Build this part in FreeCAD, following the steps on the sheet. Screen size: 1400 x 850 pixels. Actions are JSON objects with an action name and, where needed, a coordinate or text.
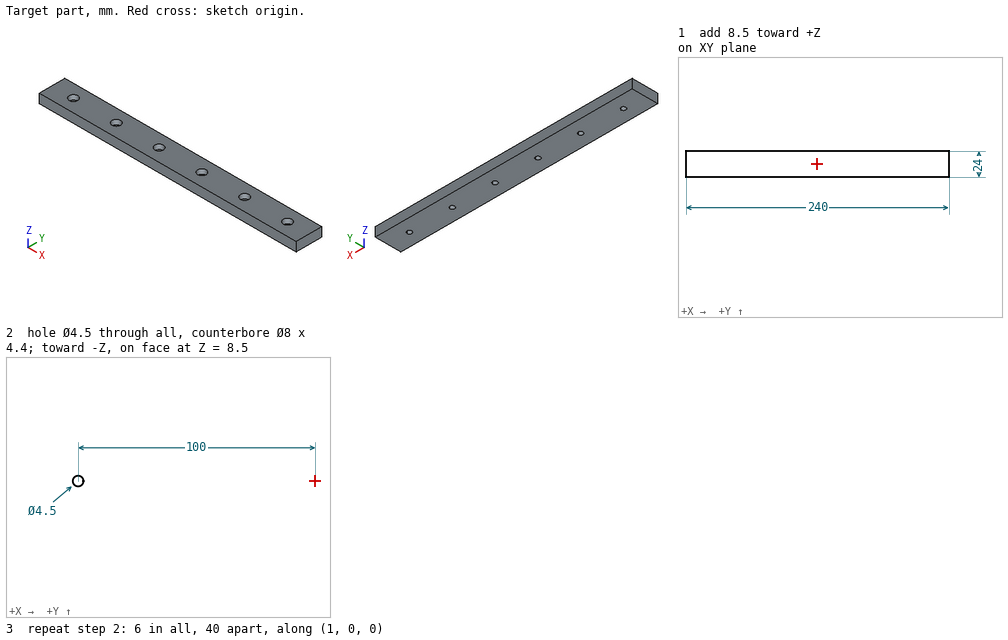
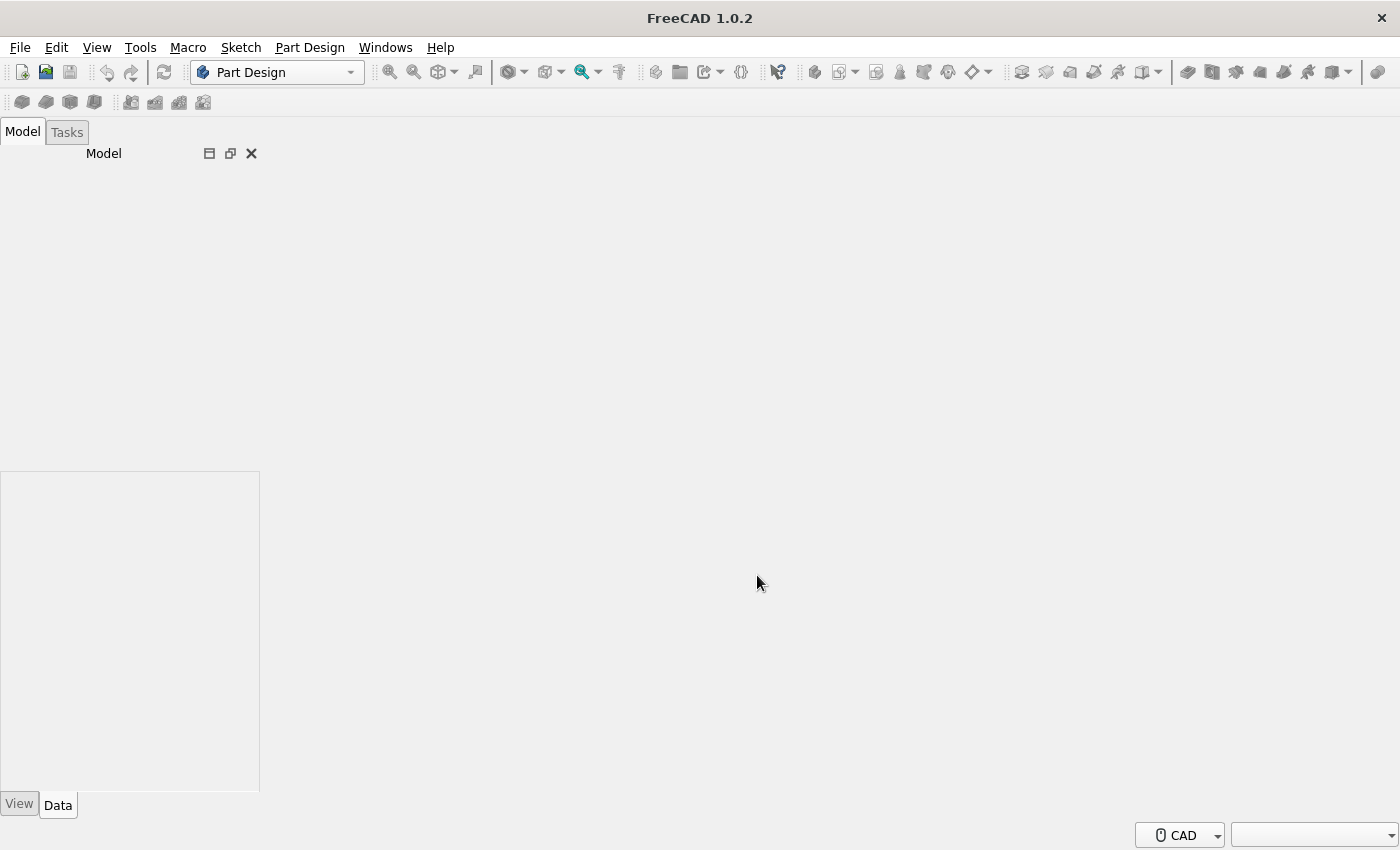
{"action": "key", "text": "ctrl+n"}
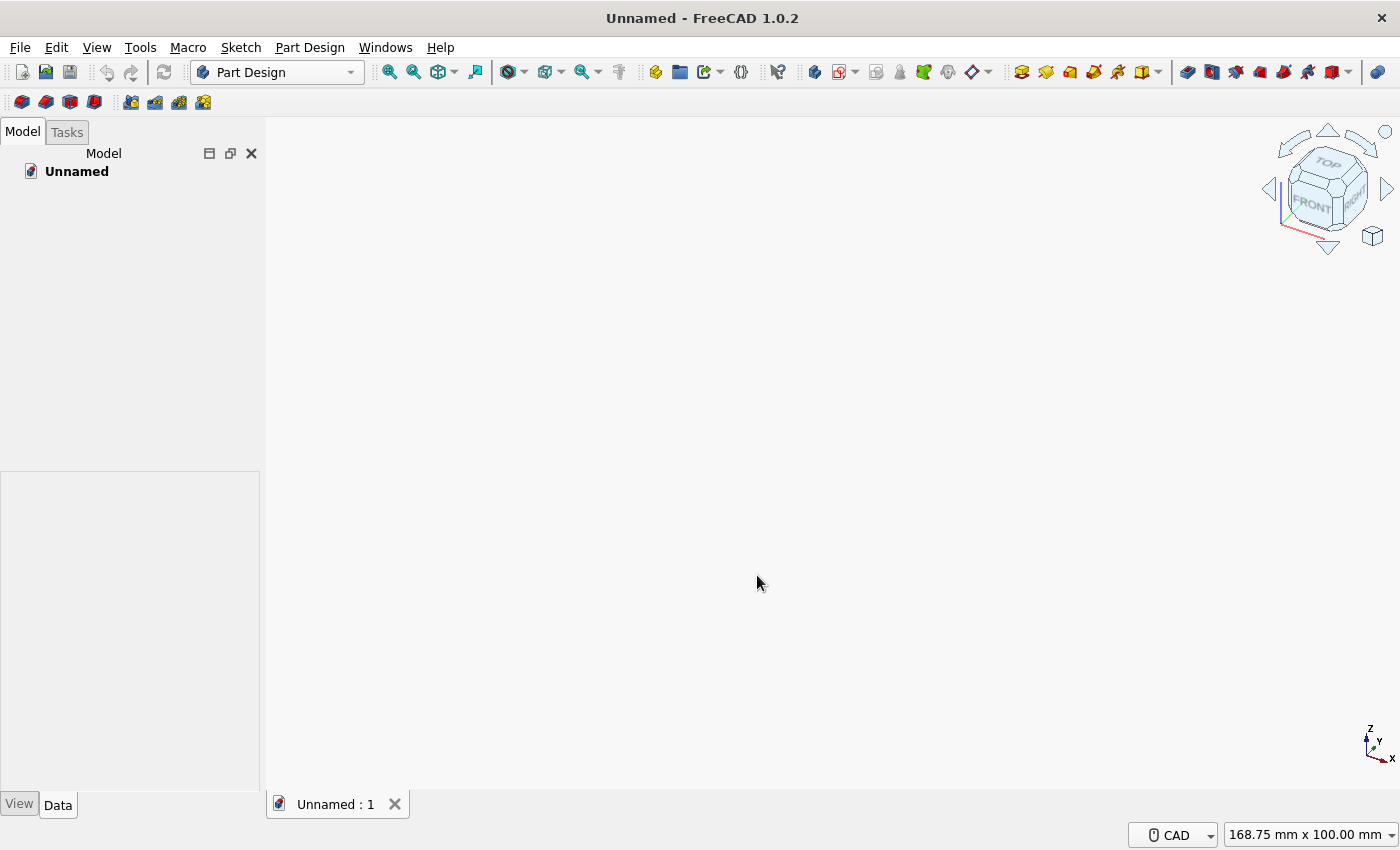
{"action": "left_click", "coordinate": [840, 72]}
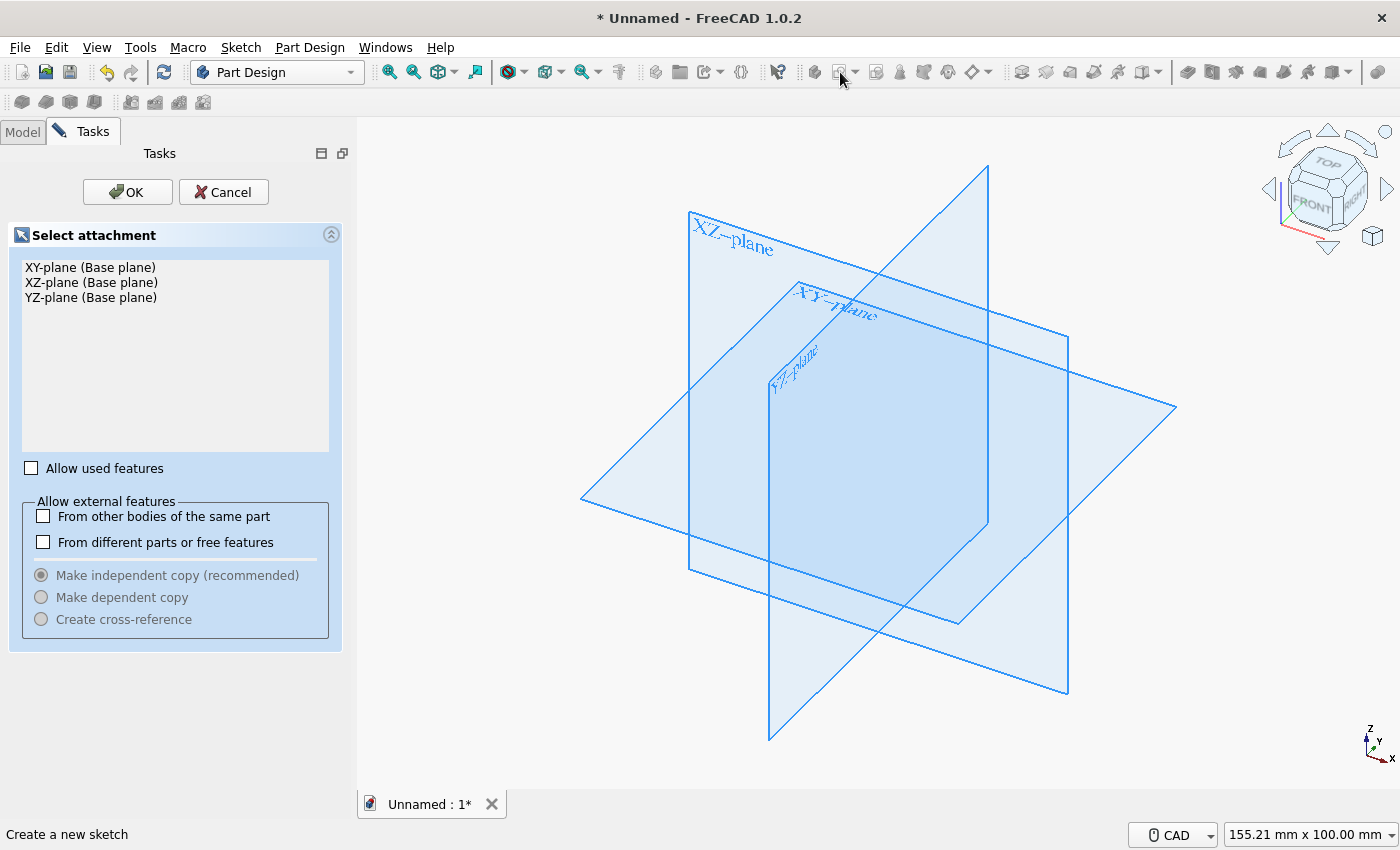
{"action": "left_click", "coordinate": [82, 268]}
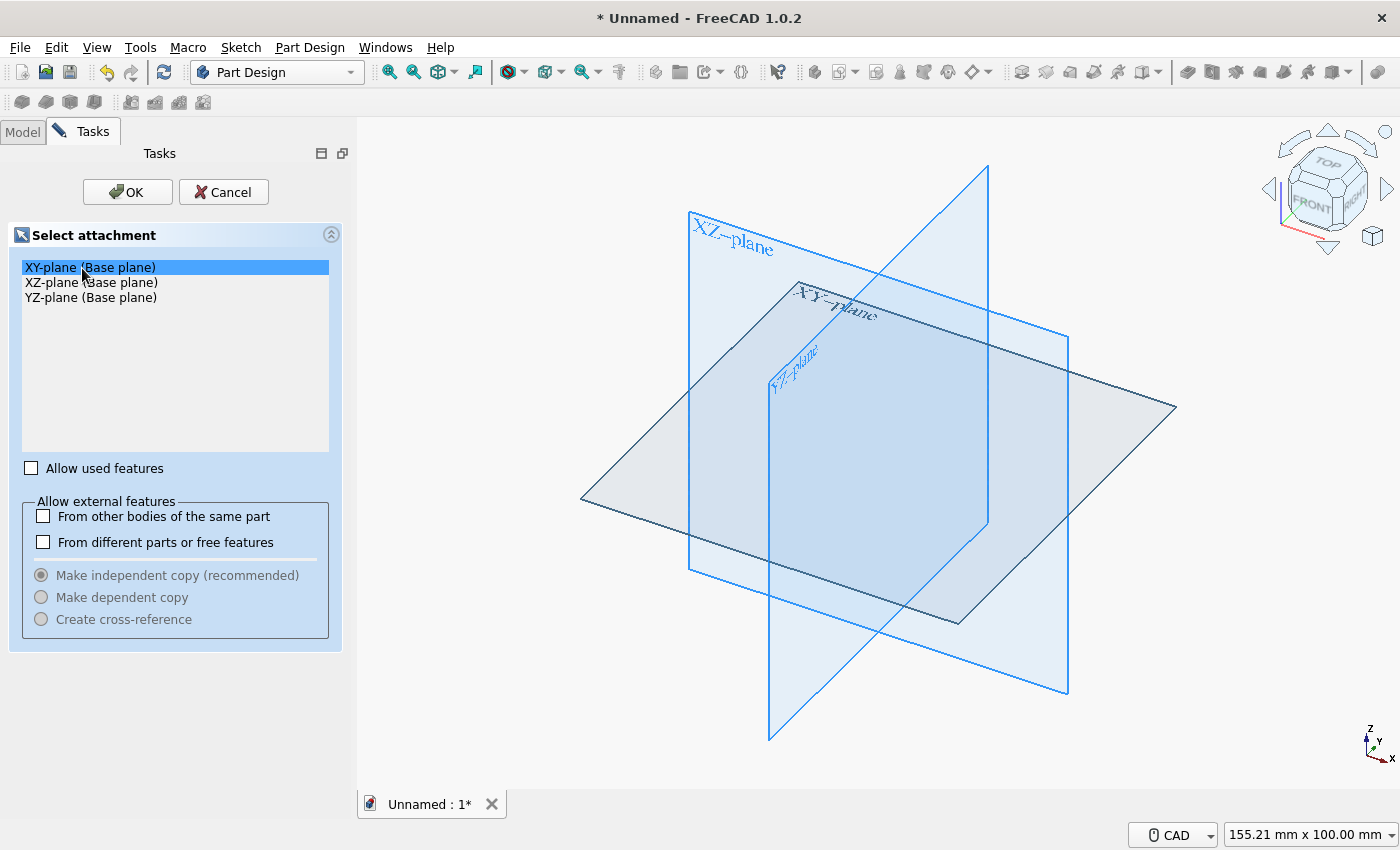
{"action": "left_click", "coordinate": [128, 192]}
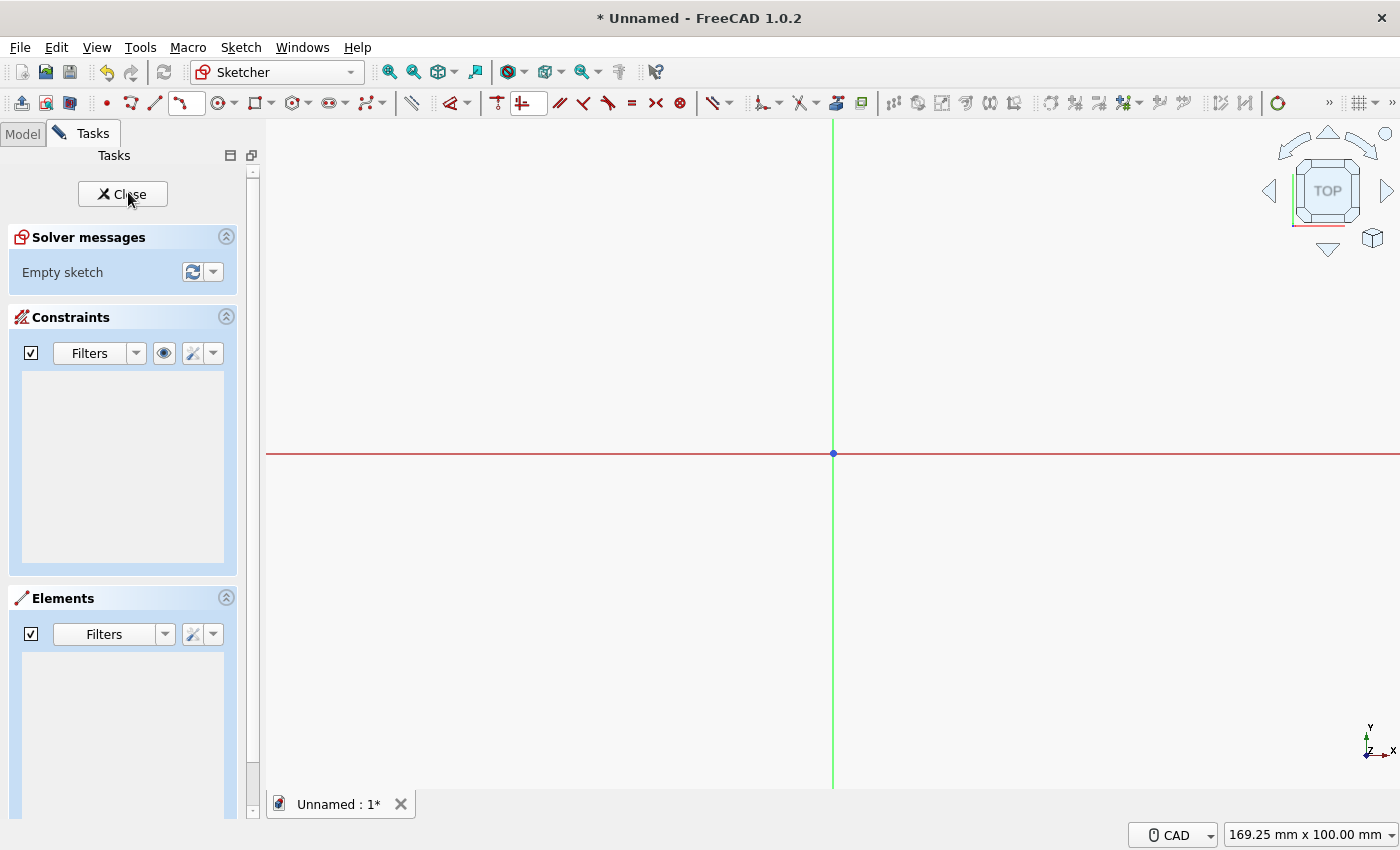
{"action": "scroll", "coordinate": [709, 454], "scroll_direction": "down", "scroll_amount": 4}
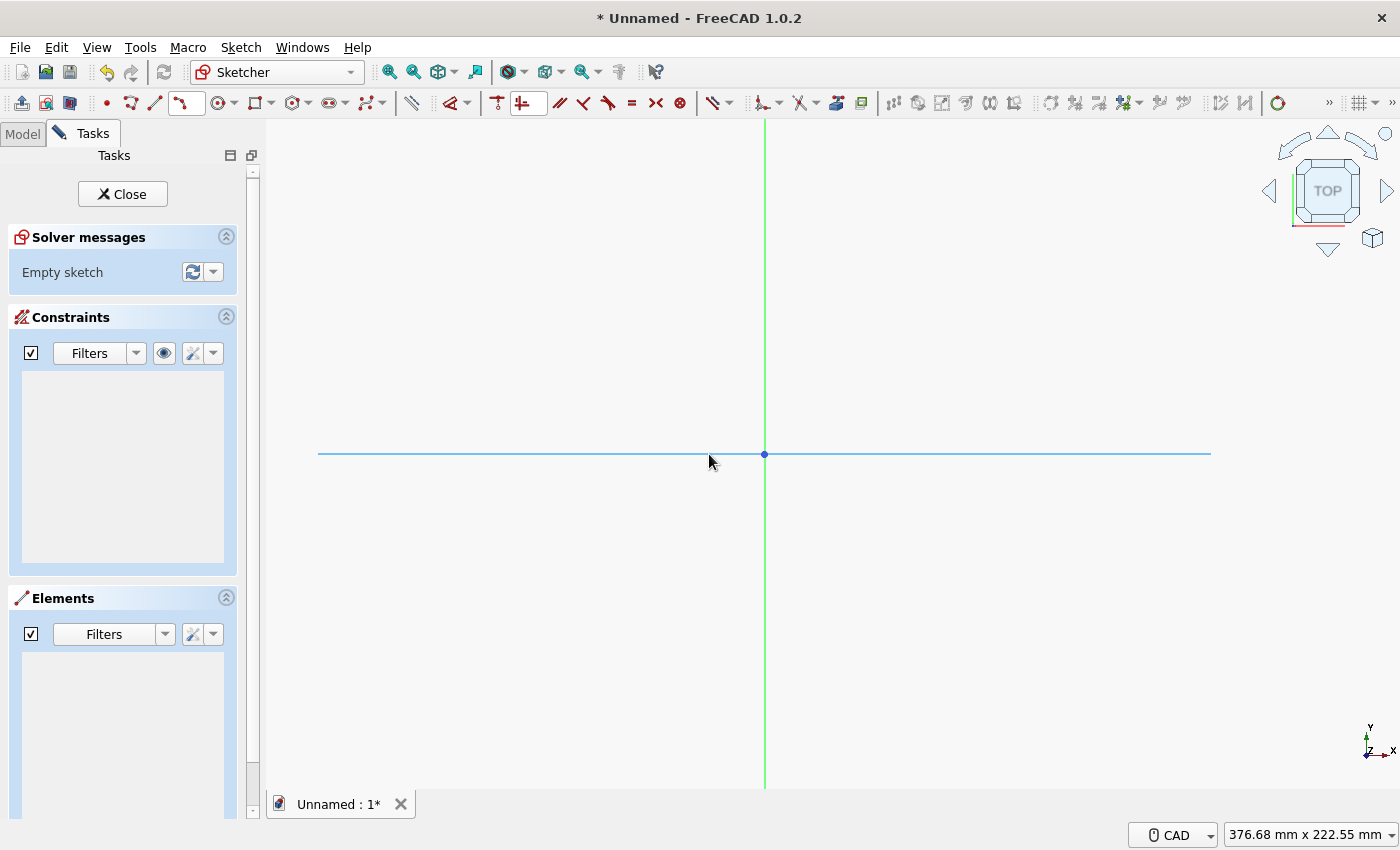
{"action": "left_click", "coordinate": [274, 104]}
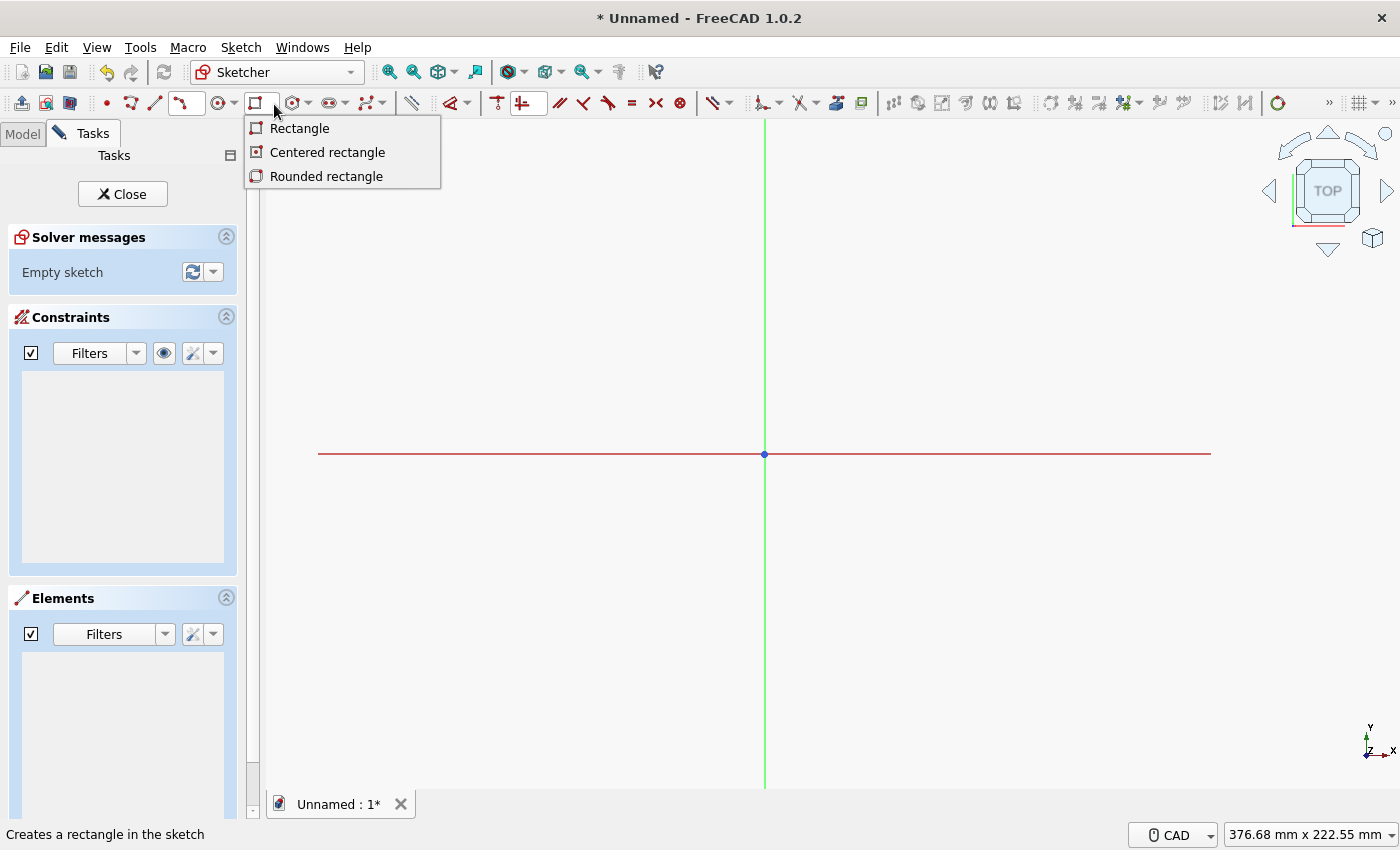
{"action": "left_click", "coordinate": [342, 152]}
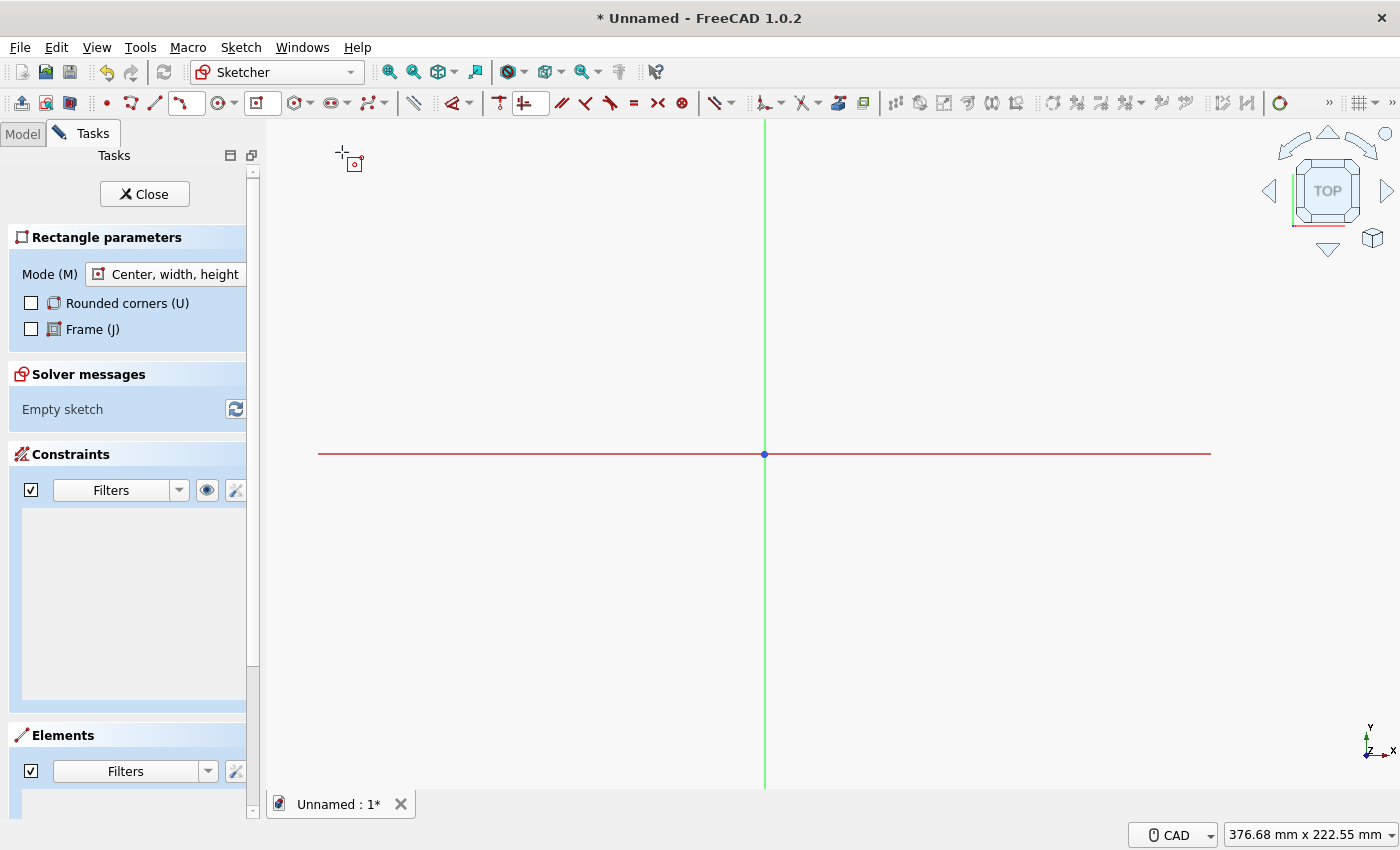
{"action": "left_click", "coordinate": [765, 454]}
{"action": "mouse_move", "coordinate": [1126, 418]}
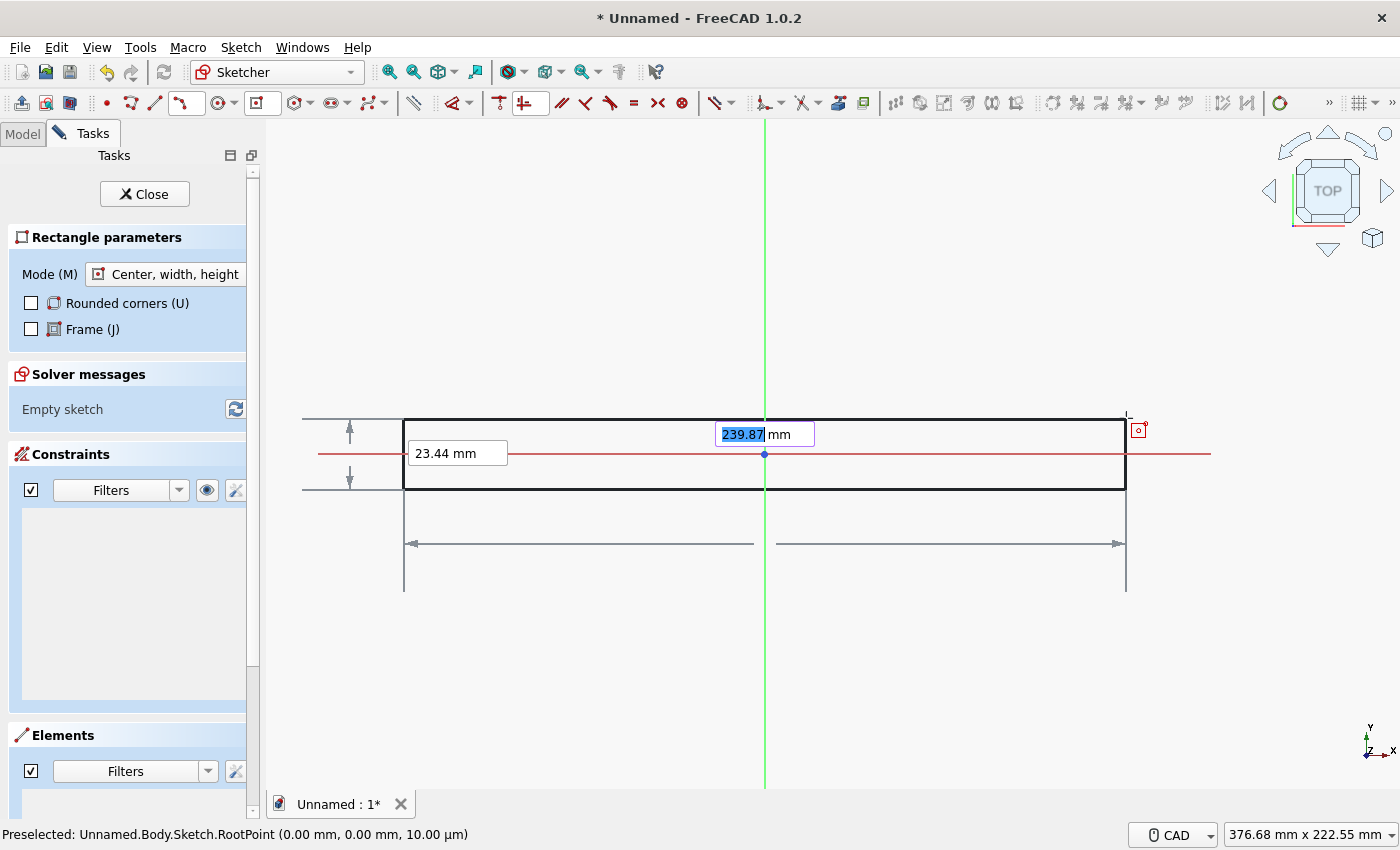
{"action": "type", "text": "240"}
{"action": "key", "text": "Tab"}
{"action": "type", "text": "24"}
{"action": "key", "text": "Return"}
{"action": "key", "text": "Escape"}